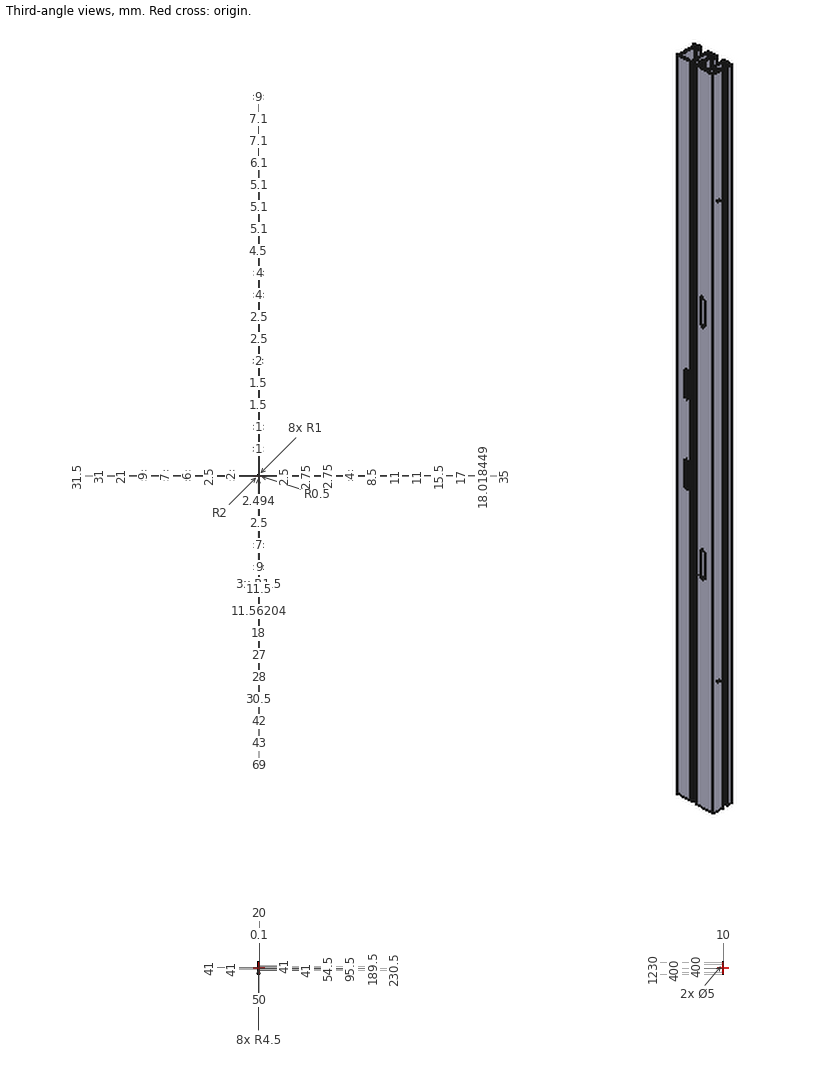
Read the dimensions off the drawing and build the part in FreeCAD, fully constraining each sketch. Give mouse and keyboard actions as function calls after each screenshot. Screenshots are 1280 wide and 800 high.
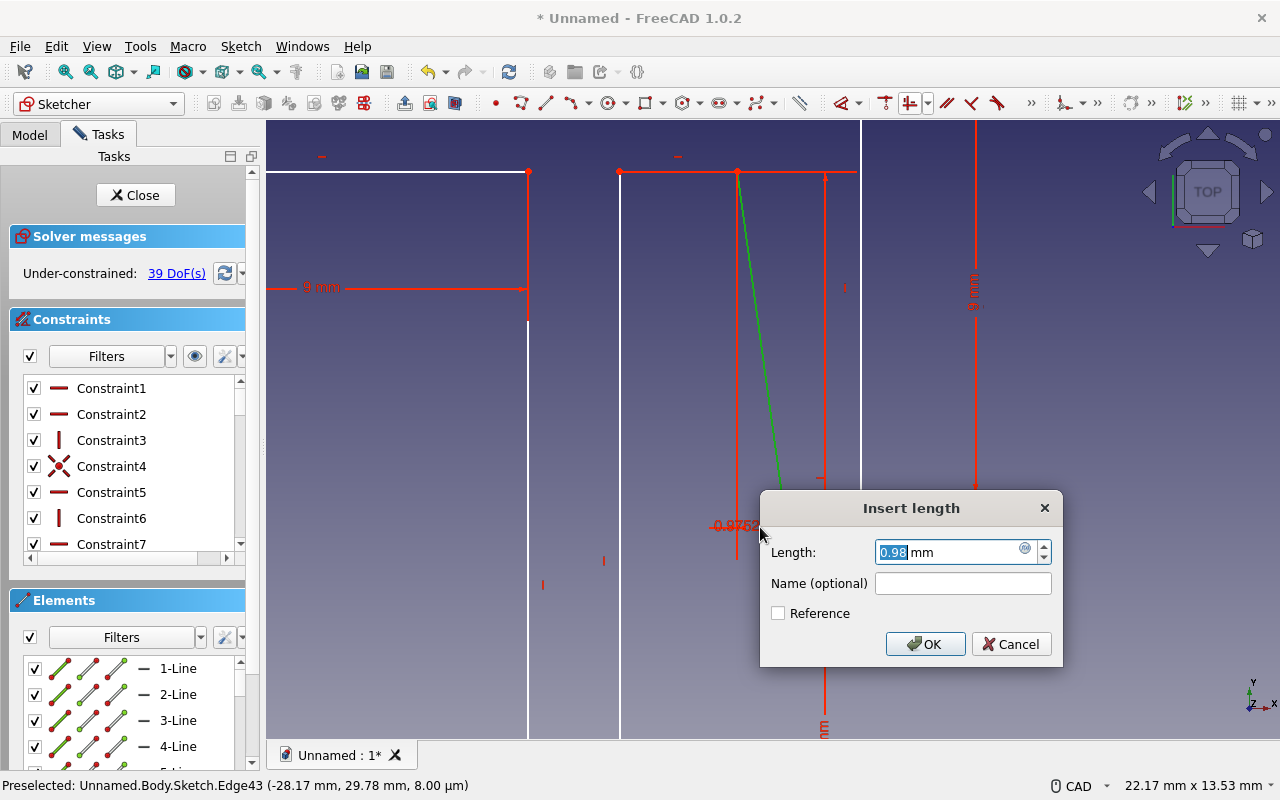
text(1)
key(Return)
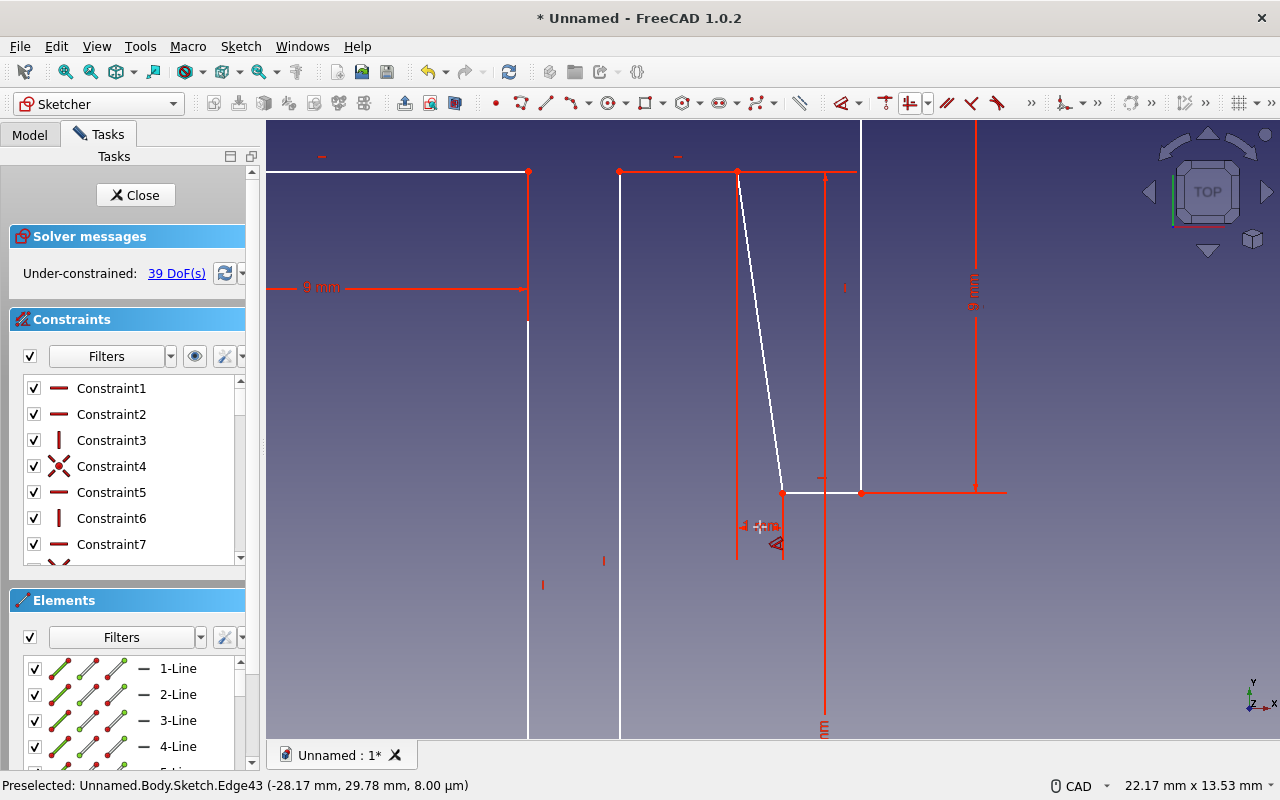
scroll(757, 350, down, 9)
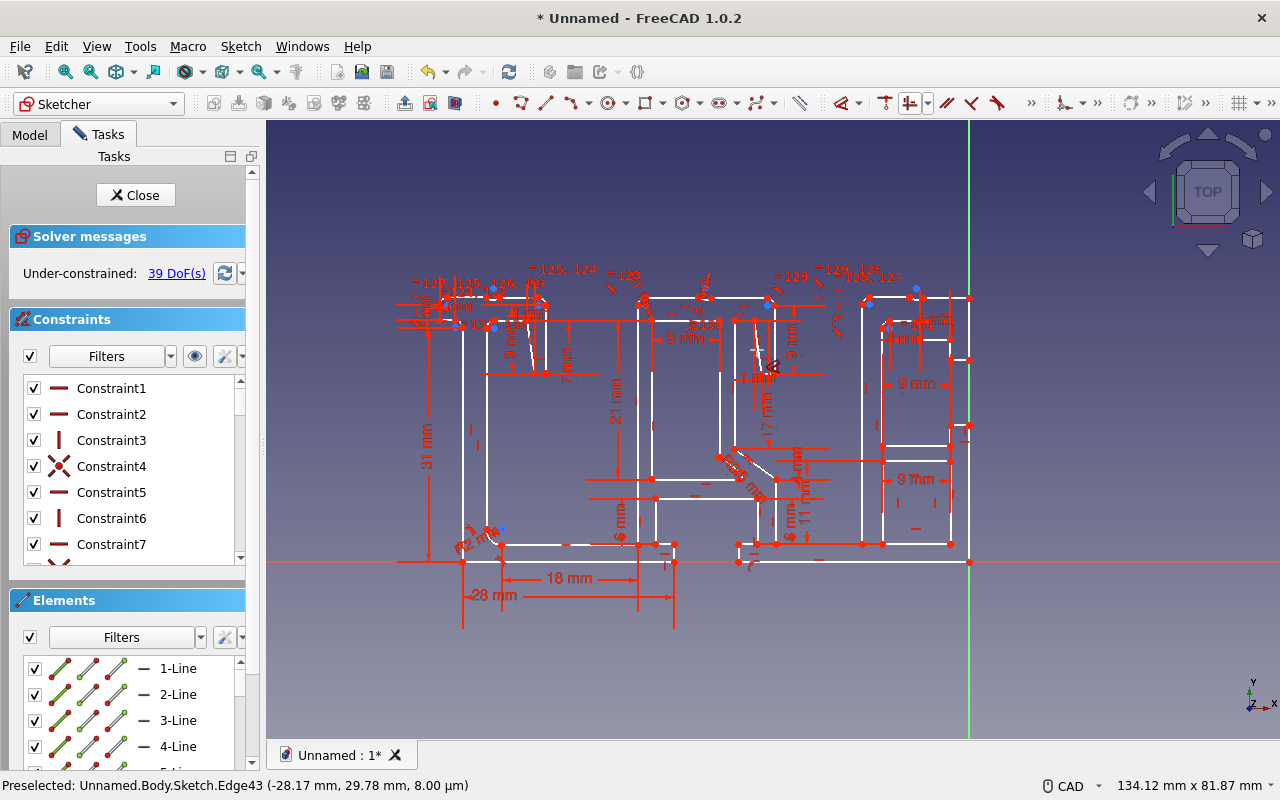
click(756, 337)
click(844, 366)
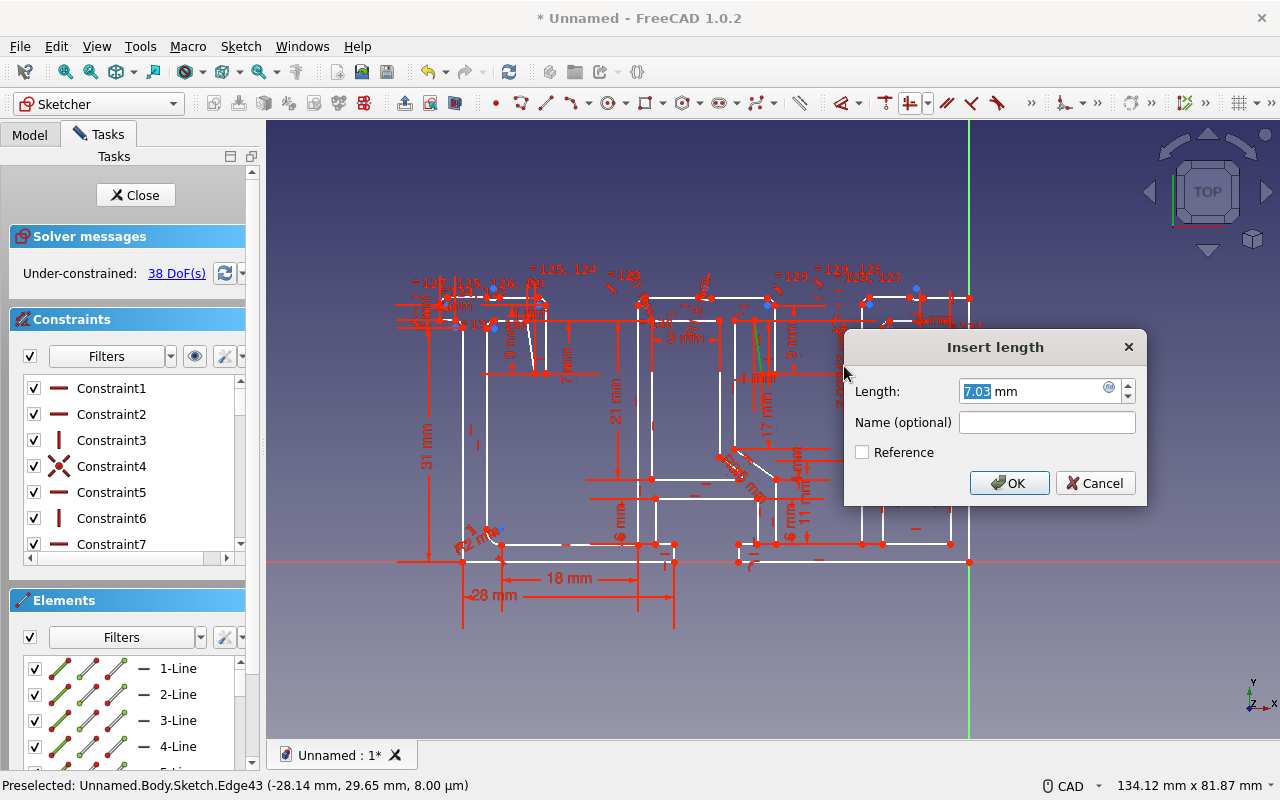
text(7)
key(Return)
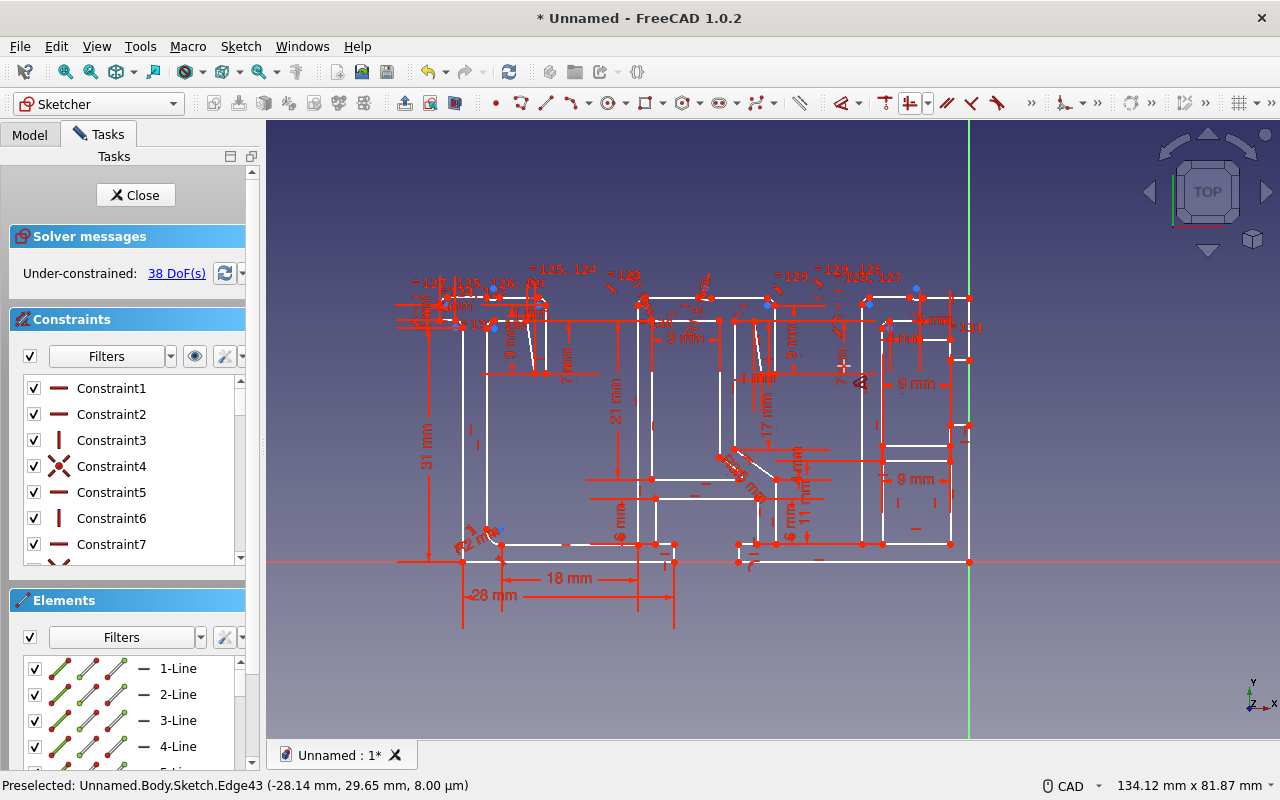
click(917, 289)
click(943, 255)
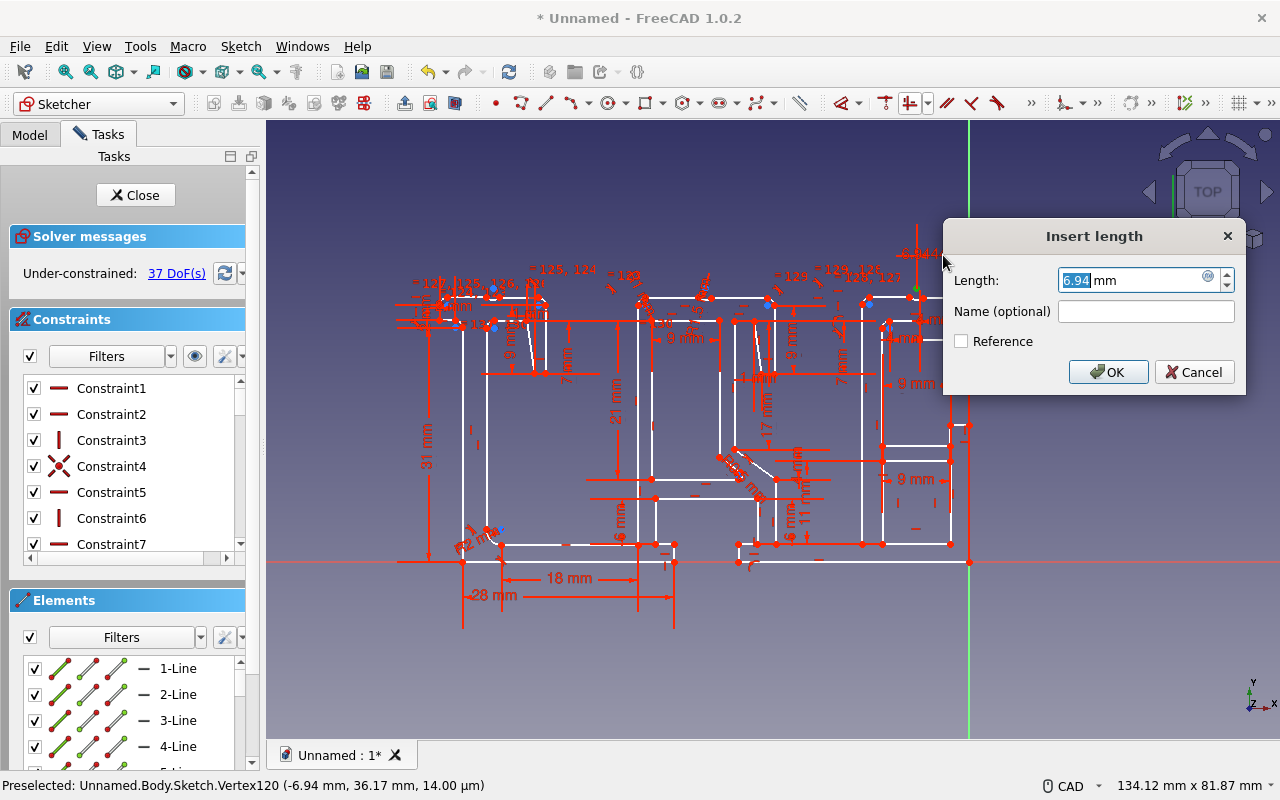
text(7)
key(Return)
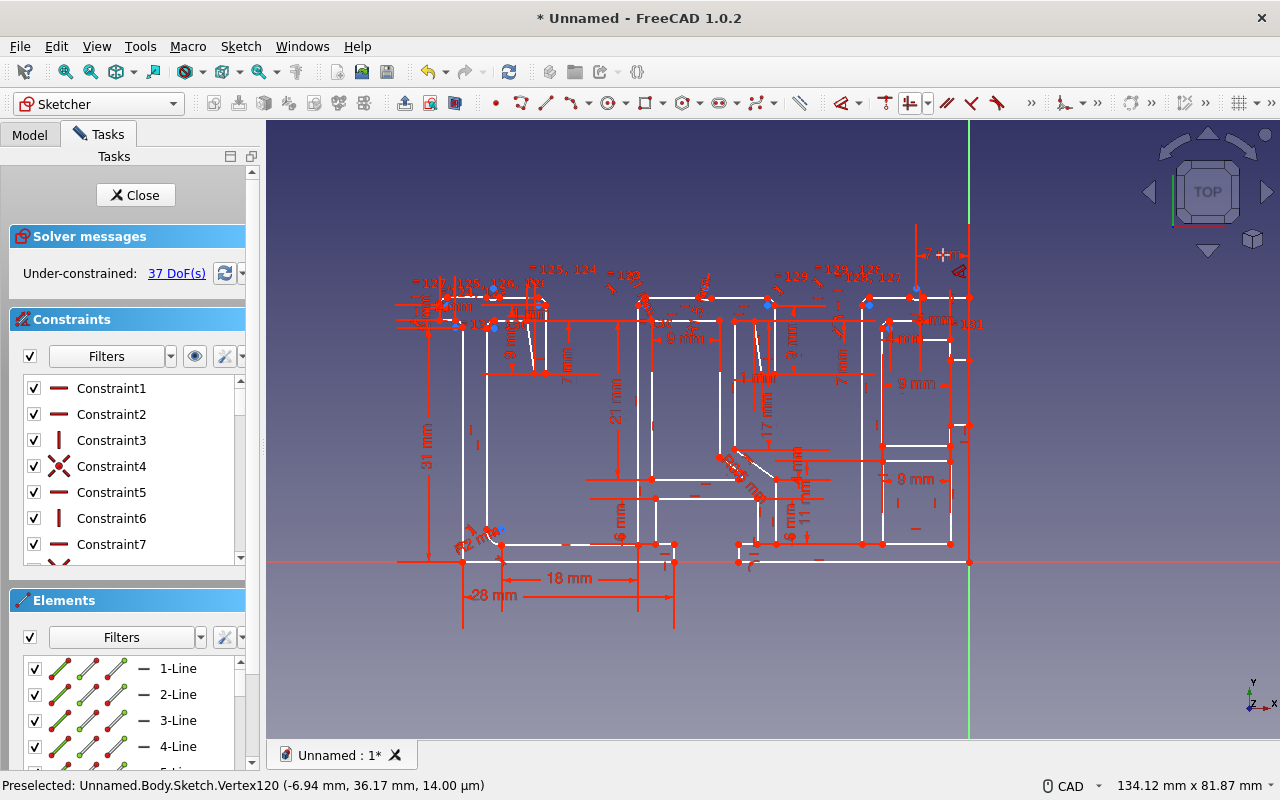
click(750, 298)
click(739, 264)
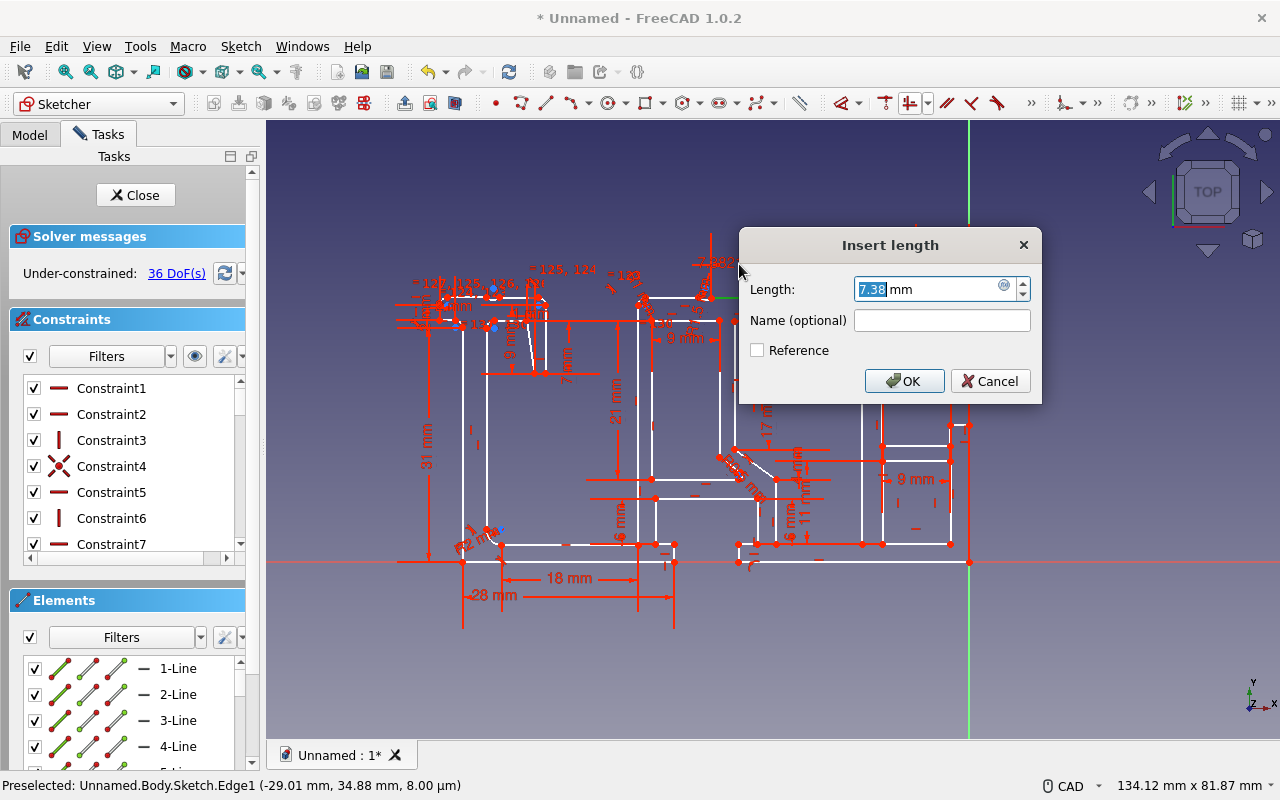
text(7.1)
key(Return)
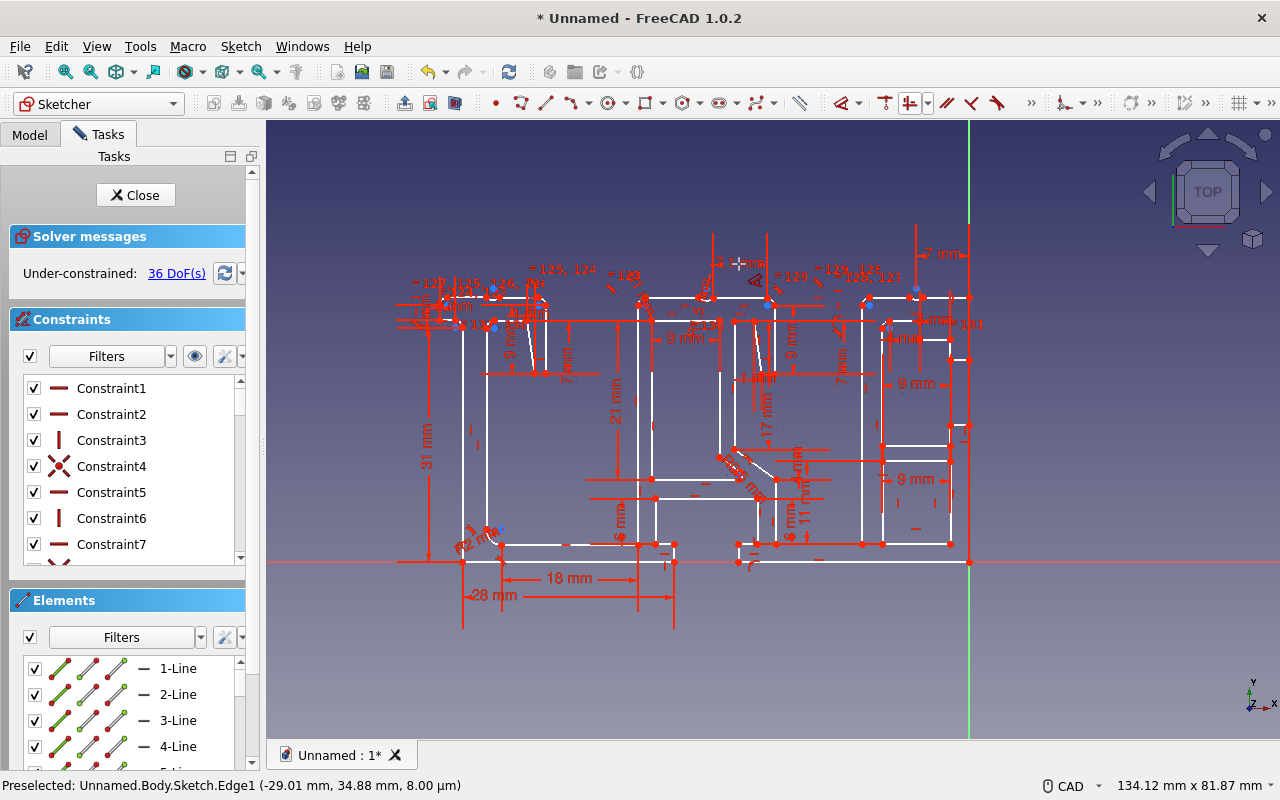
click(683, 298)
click(660, 264)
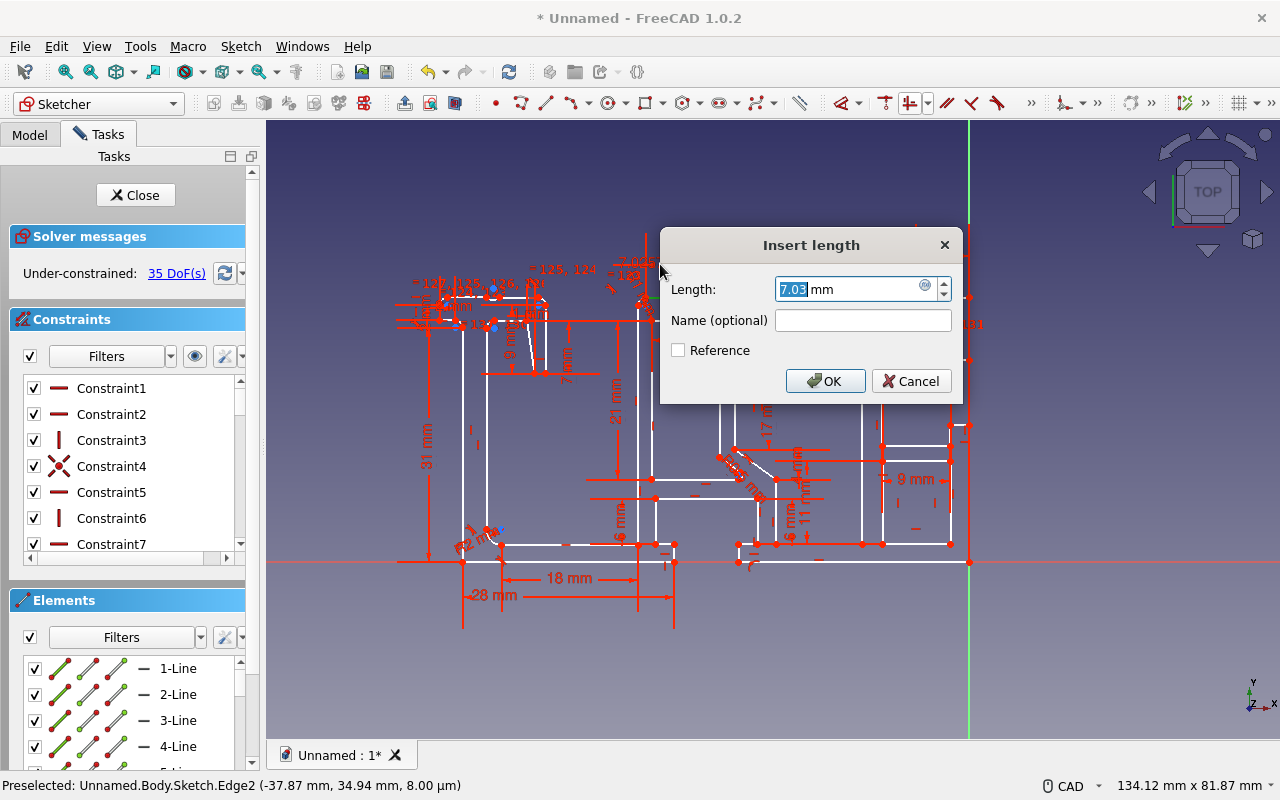
text(7.1)
key(Return)